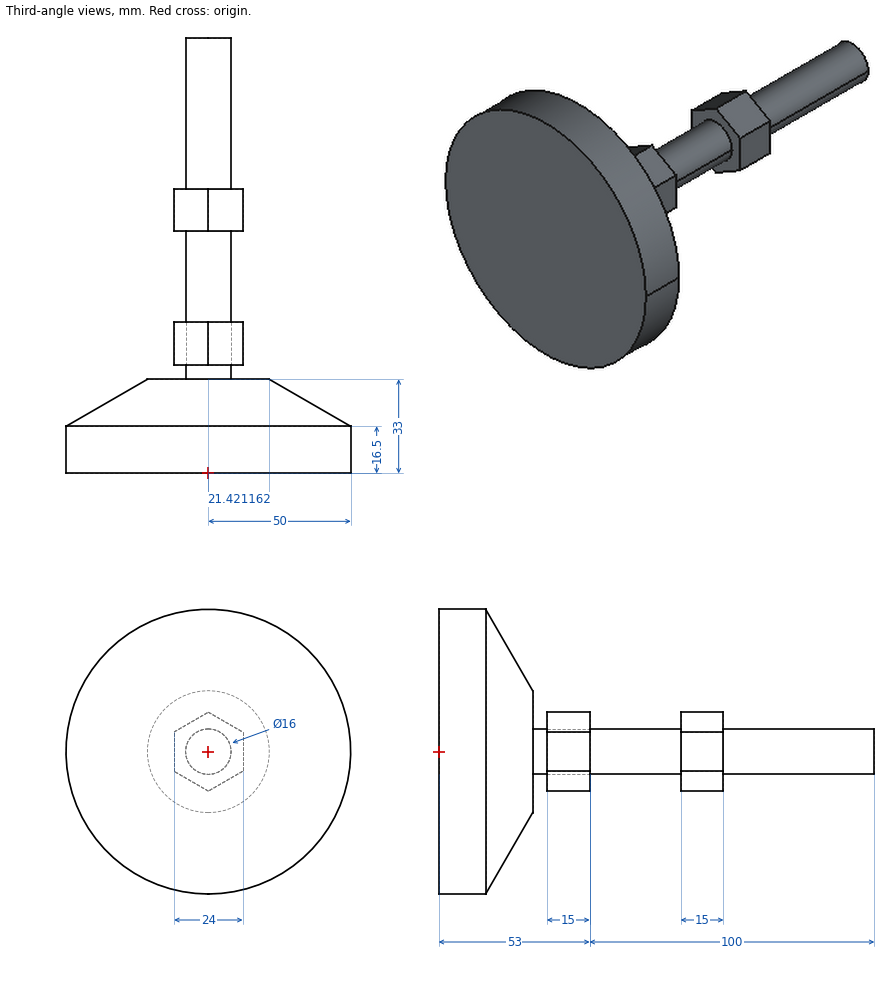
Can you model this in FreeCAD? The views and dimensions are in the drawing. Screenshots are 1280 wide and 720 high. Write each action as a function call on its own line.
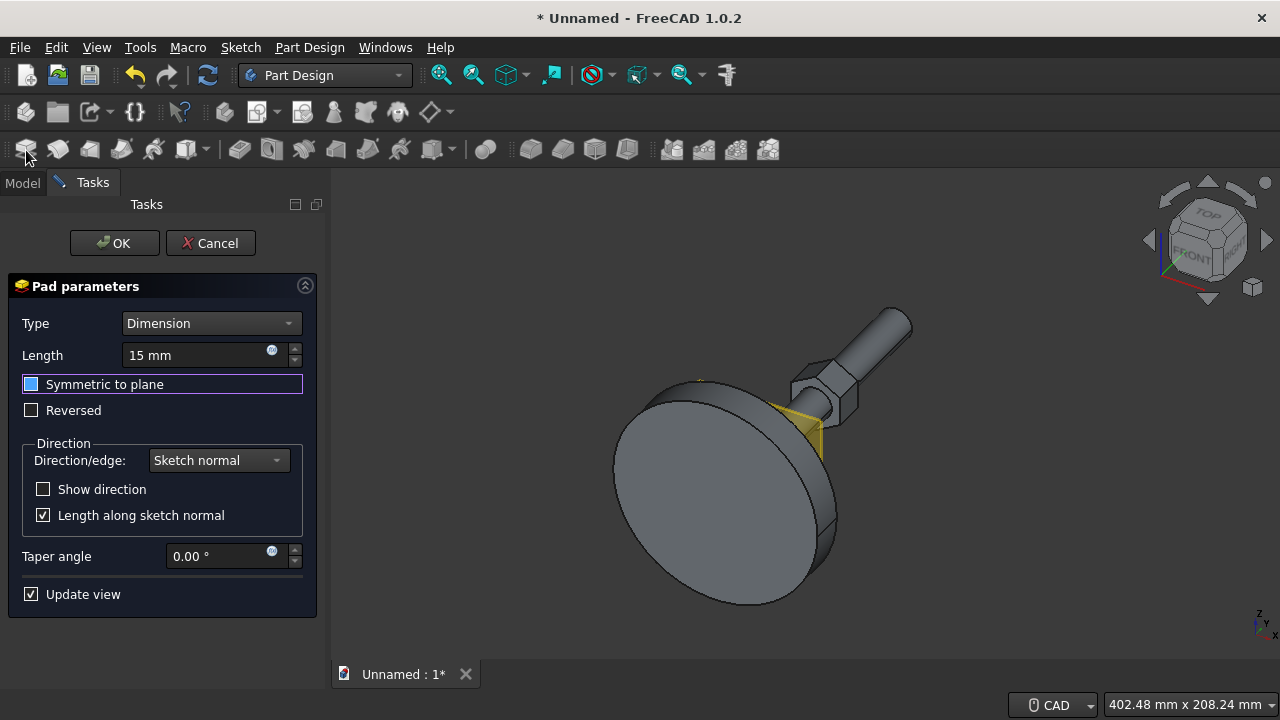
click(30, 410)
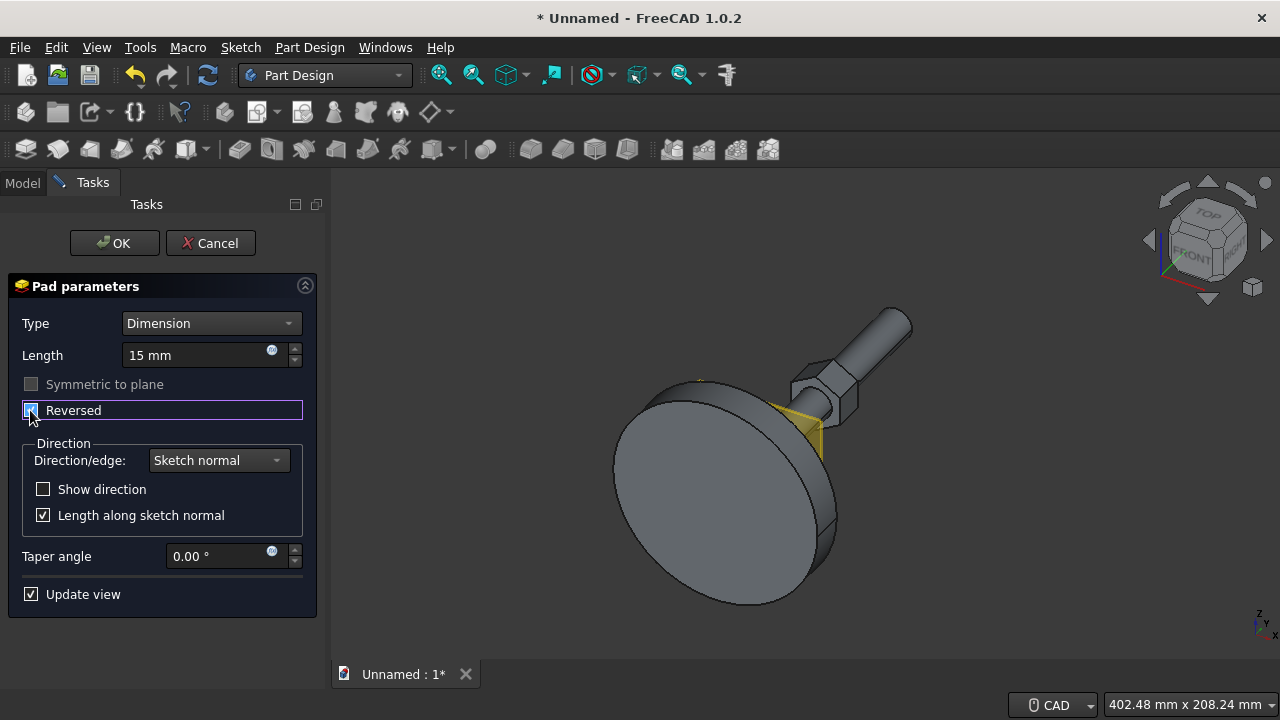
click(115, 243)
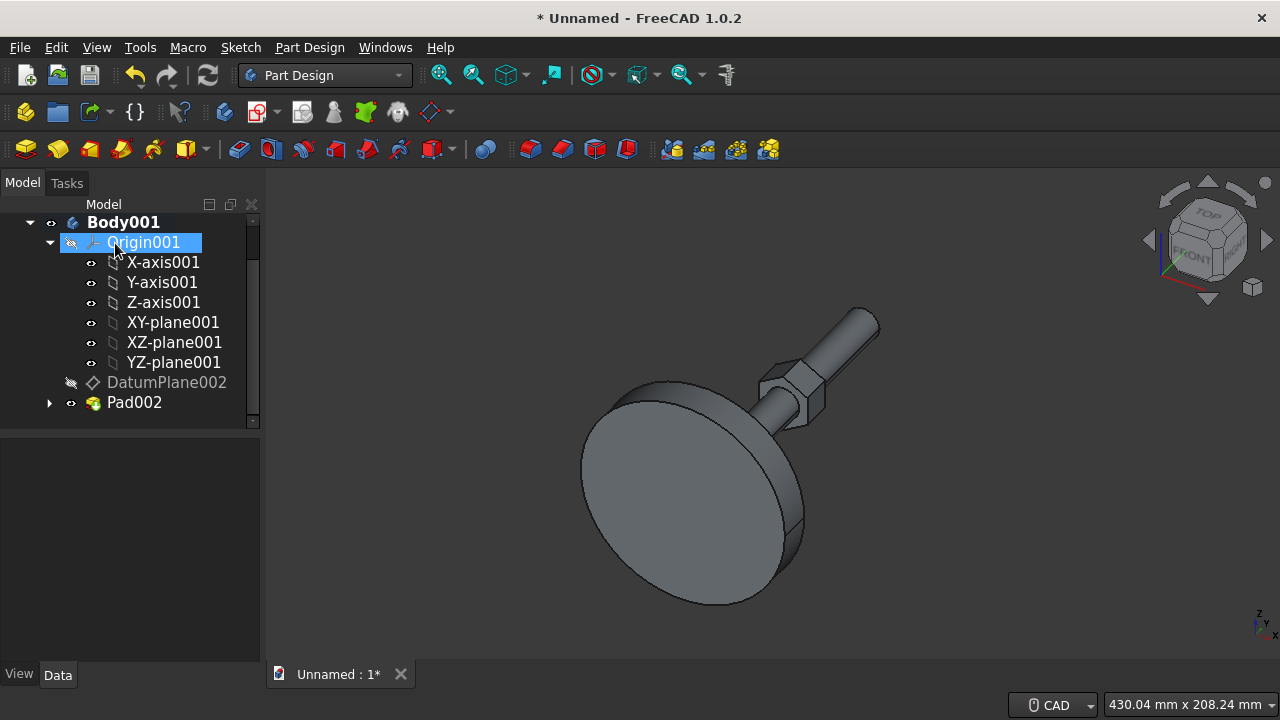
key(0)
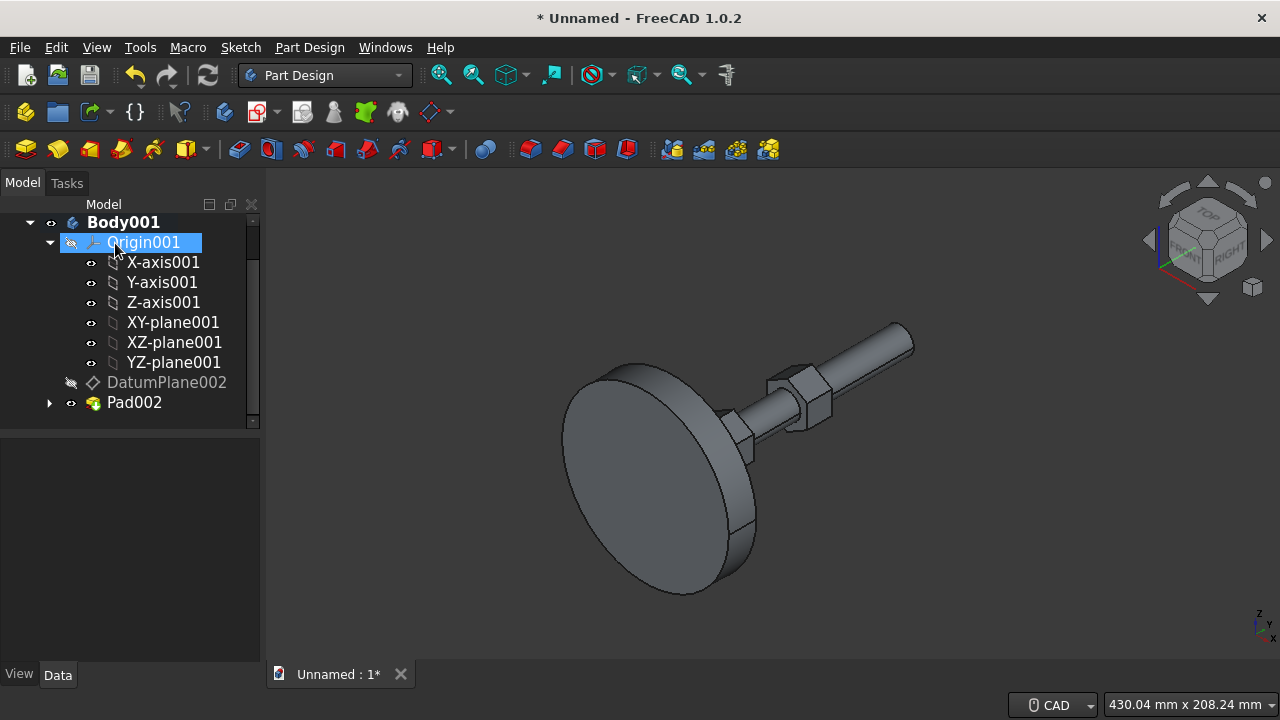
click(442, 76)